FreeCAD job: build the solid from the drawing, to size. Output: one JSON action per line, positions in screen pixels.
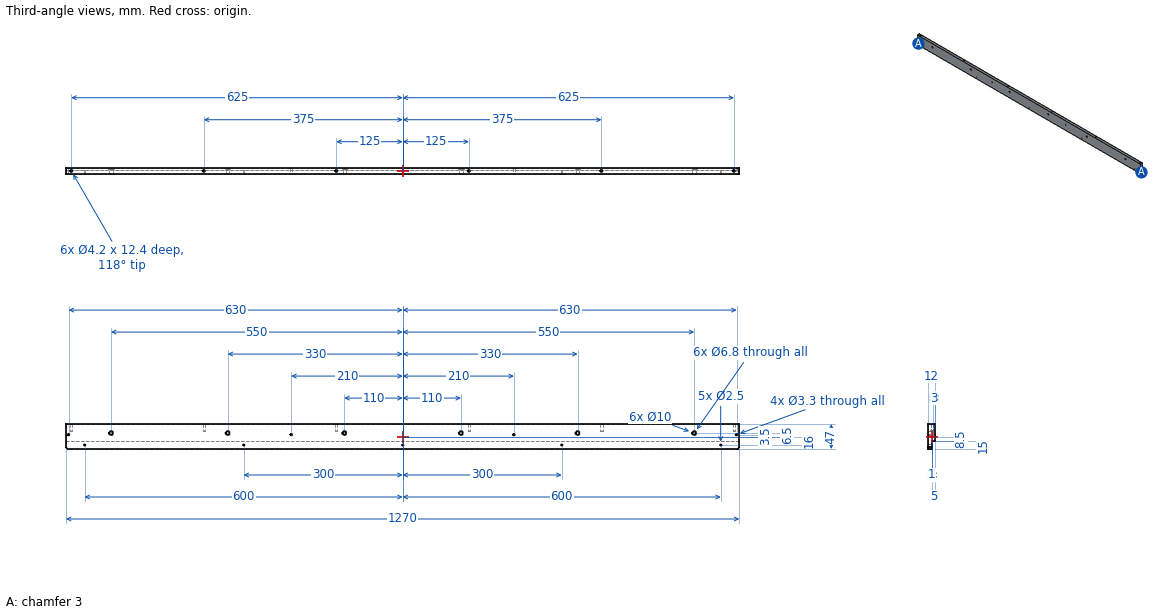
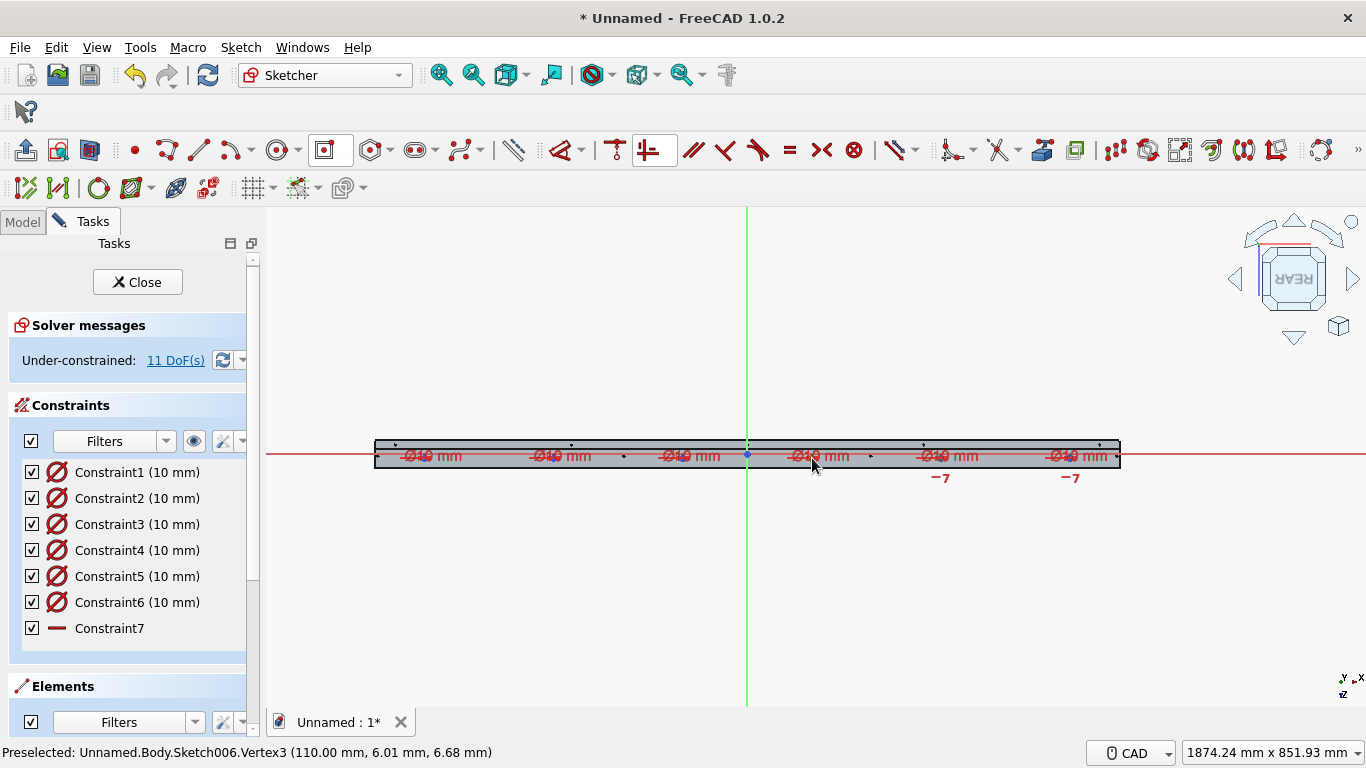
{"action": "key", "text": "h"}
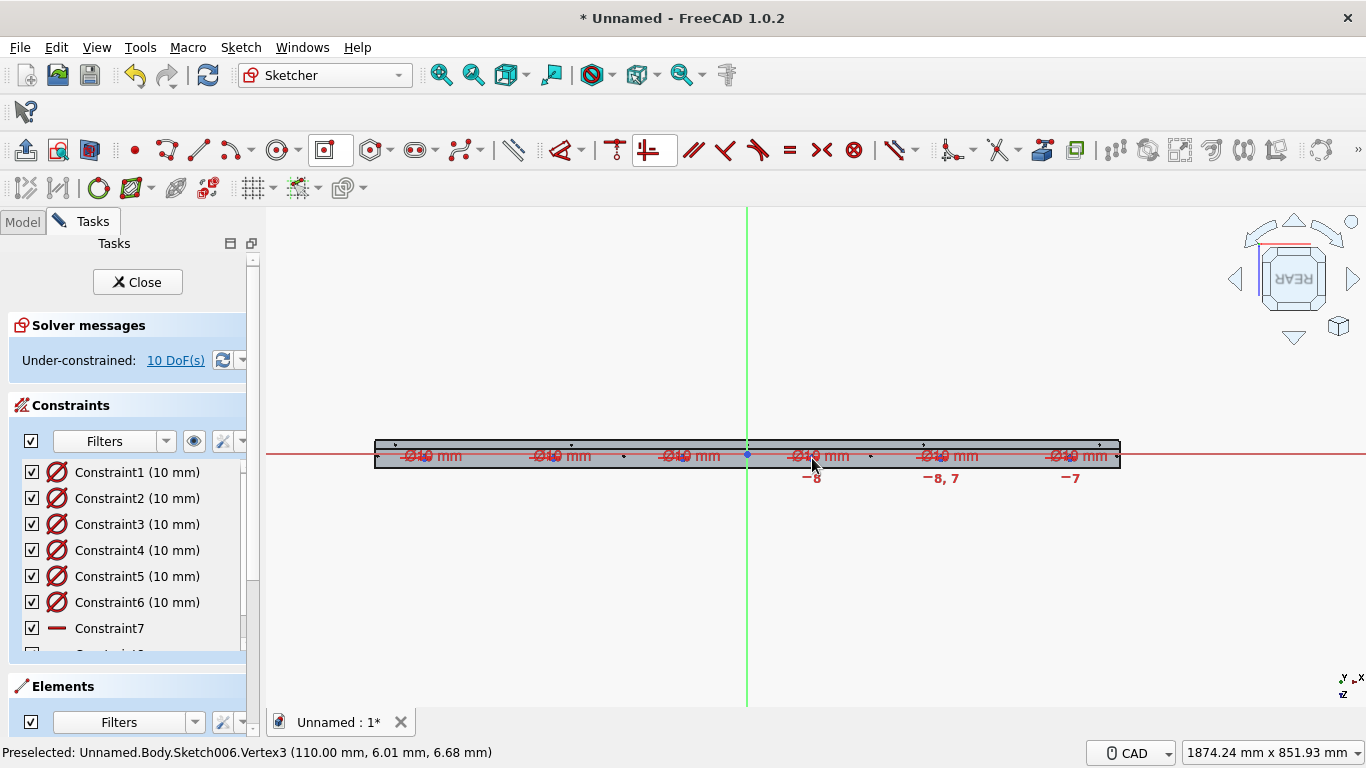
{"action": "left_click", "coordinate": [812, 458]}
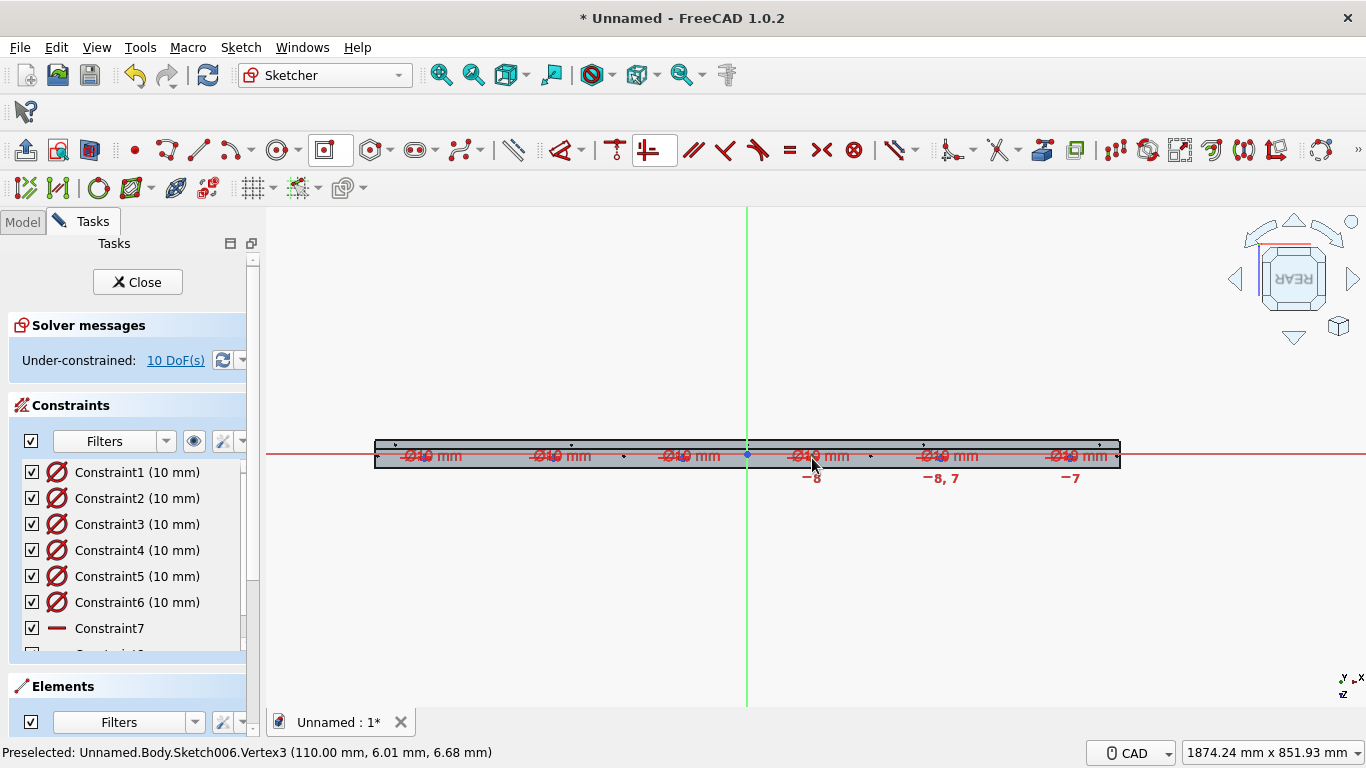
{"action": "left_click", "coordinate": [683, 458]}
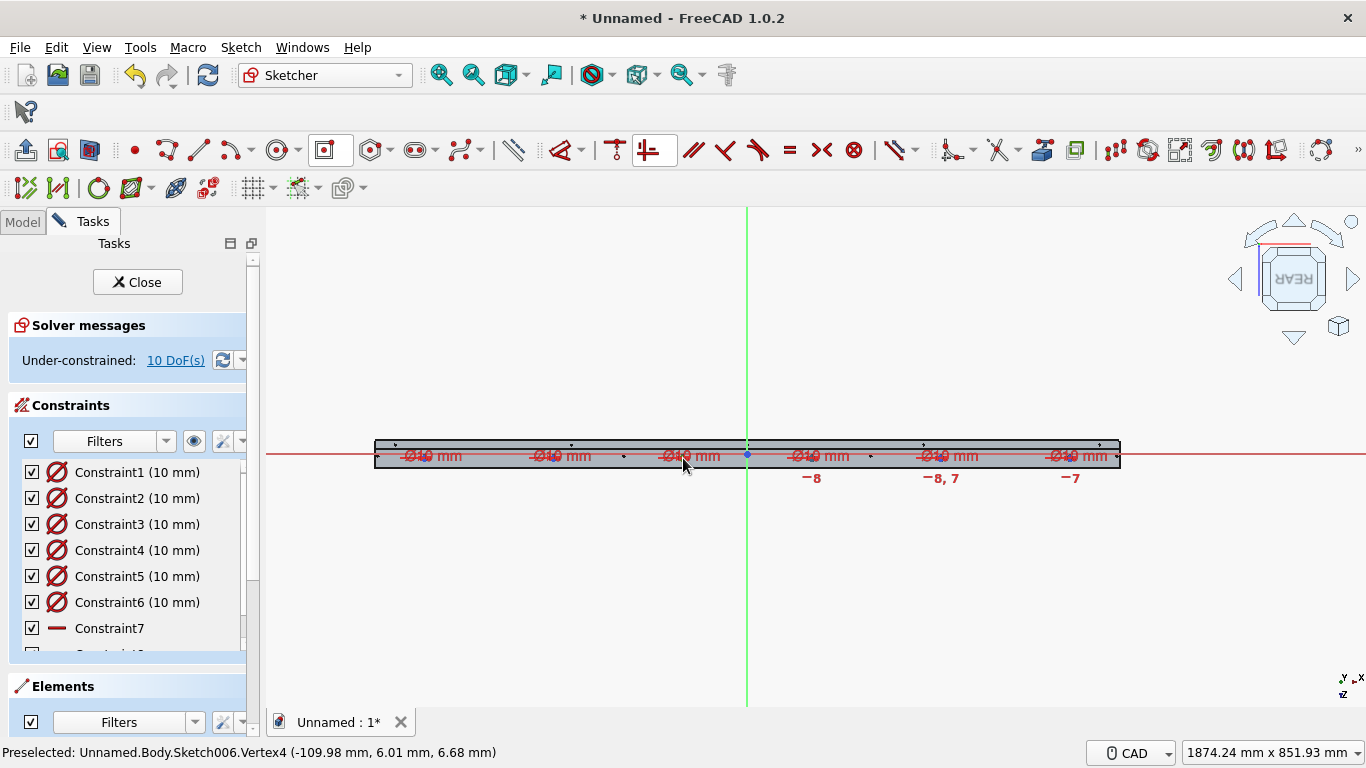
{"action": "left_click", "coordinate": [672, 150]}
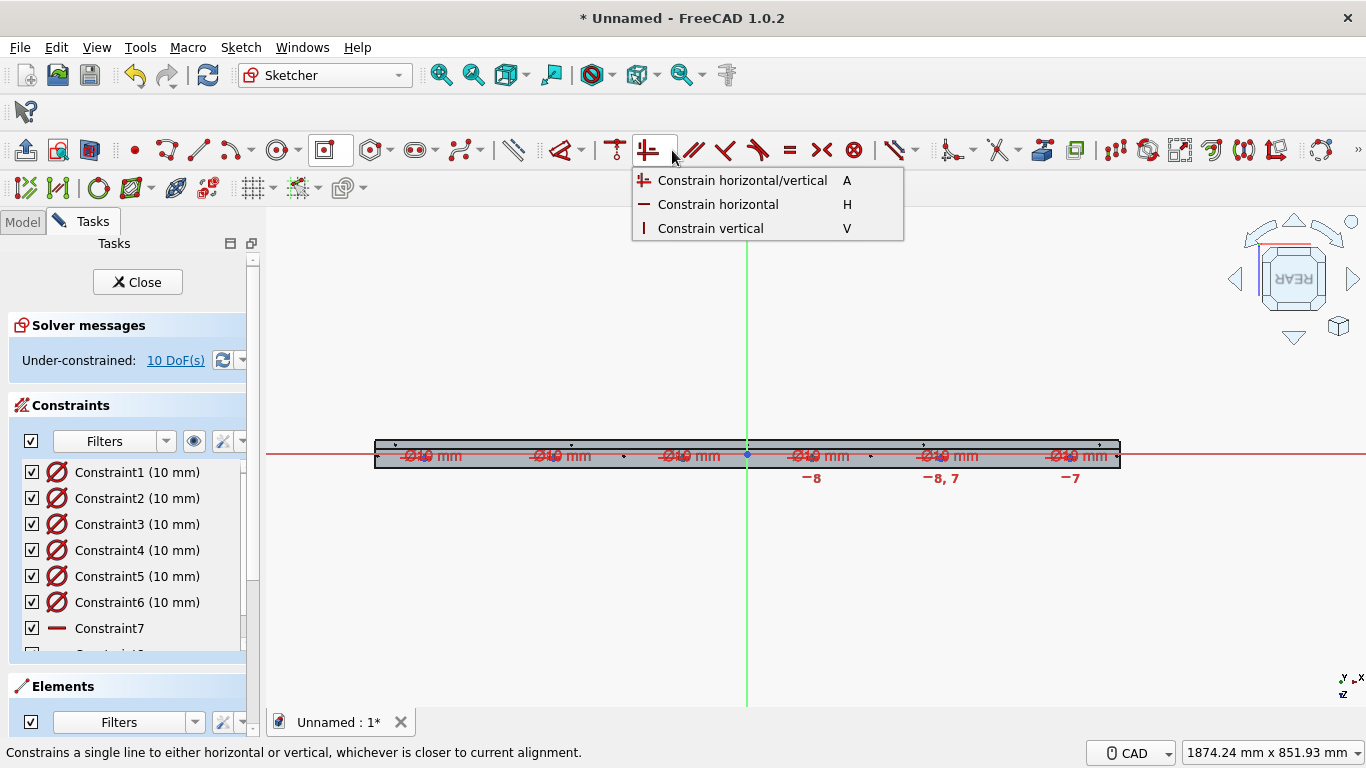
{"action": "left_click", "coordinate": [768, 204]}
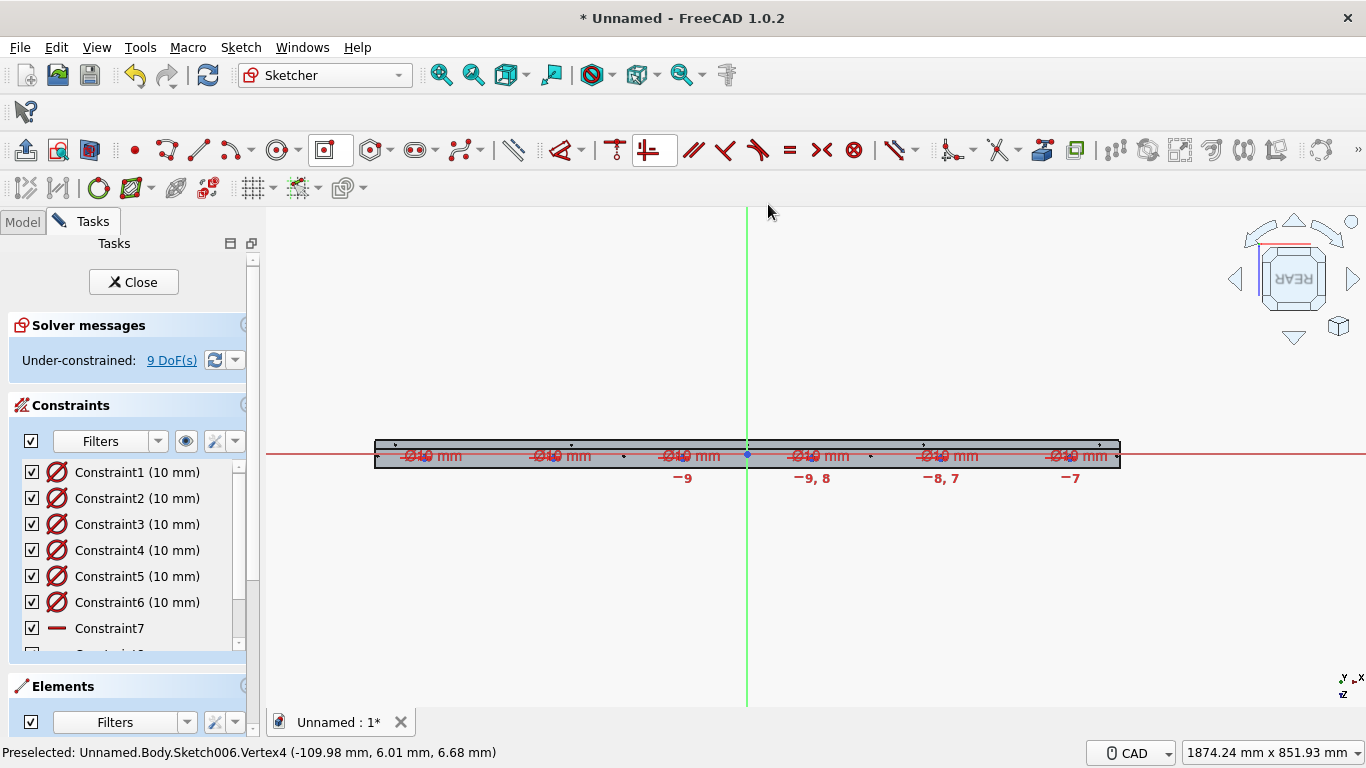
{"action": "left_click", "coordinate": [683, 458]}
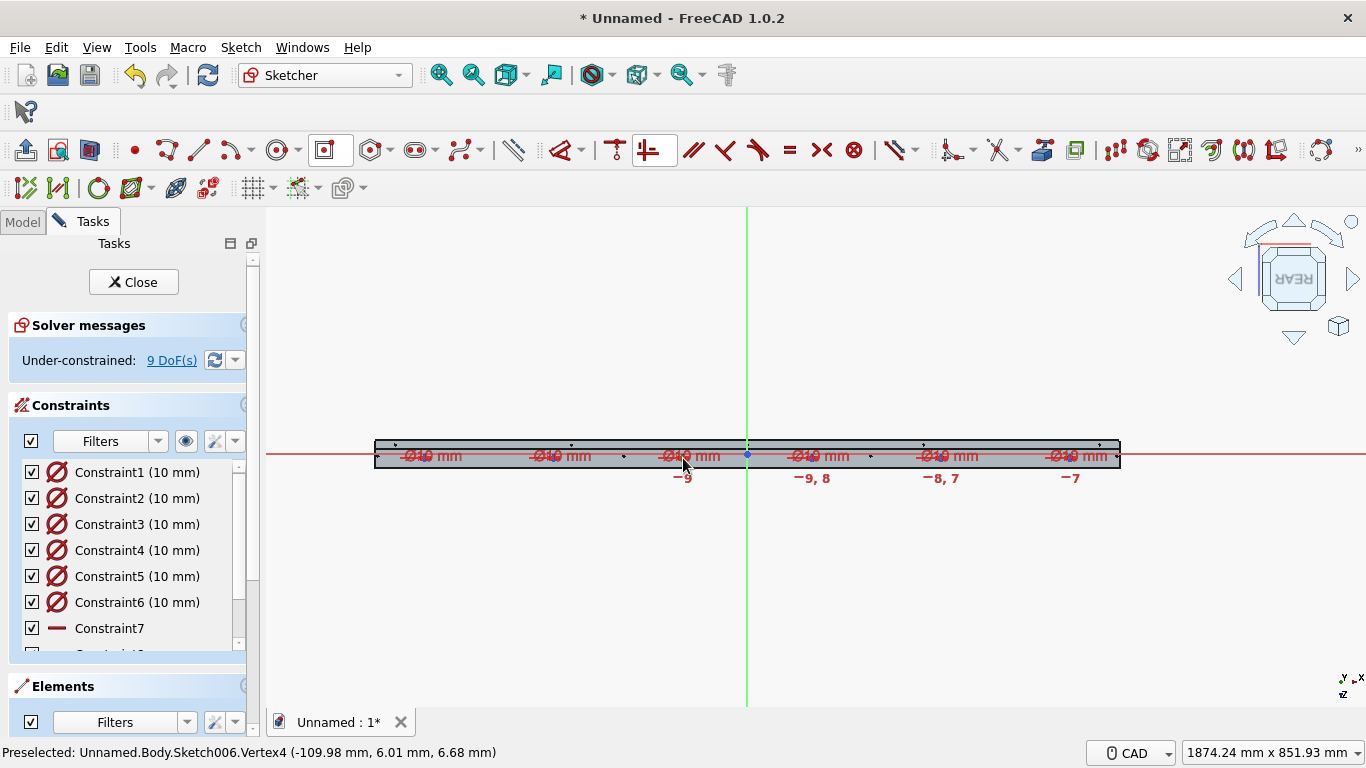
{"action": "left_click", "coordinate": [554, 458]}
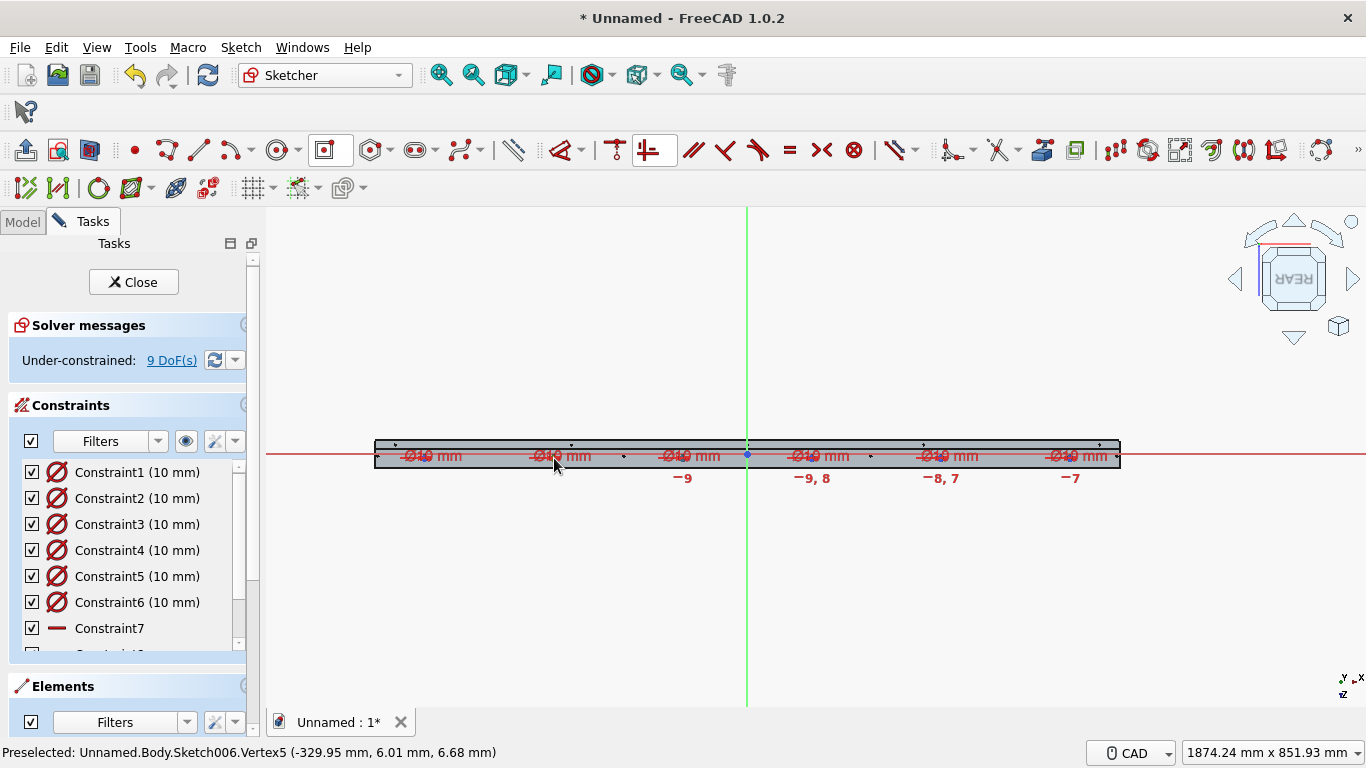
{"action": "key", "text": "h"}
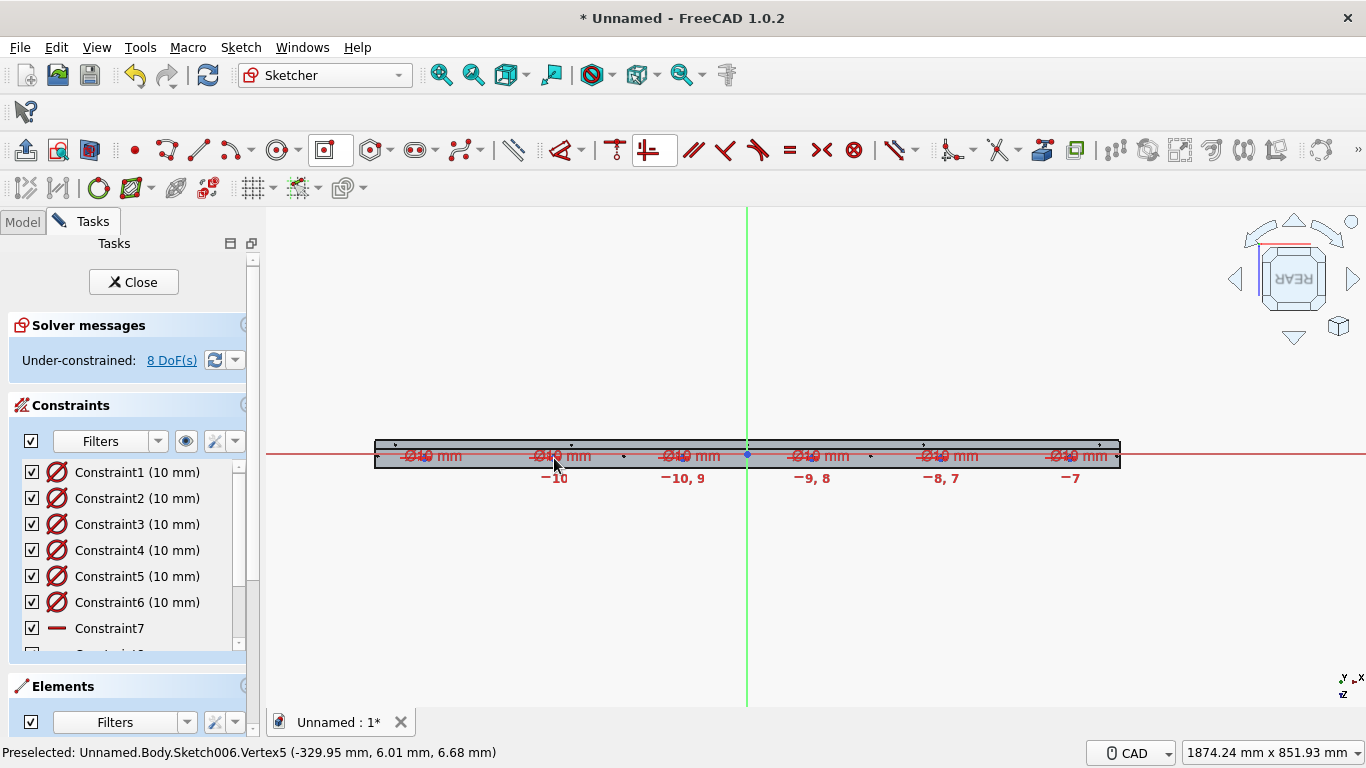
{"action": "left_click", "coordinate": [554, 458]}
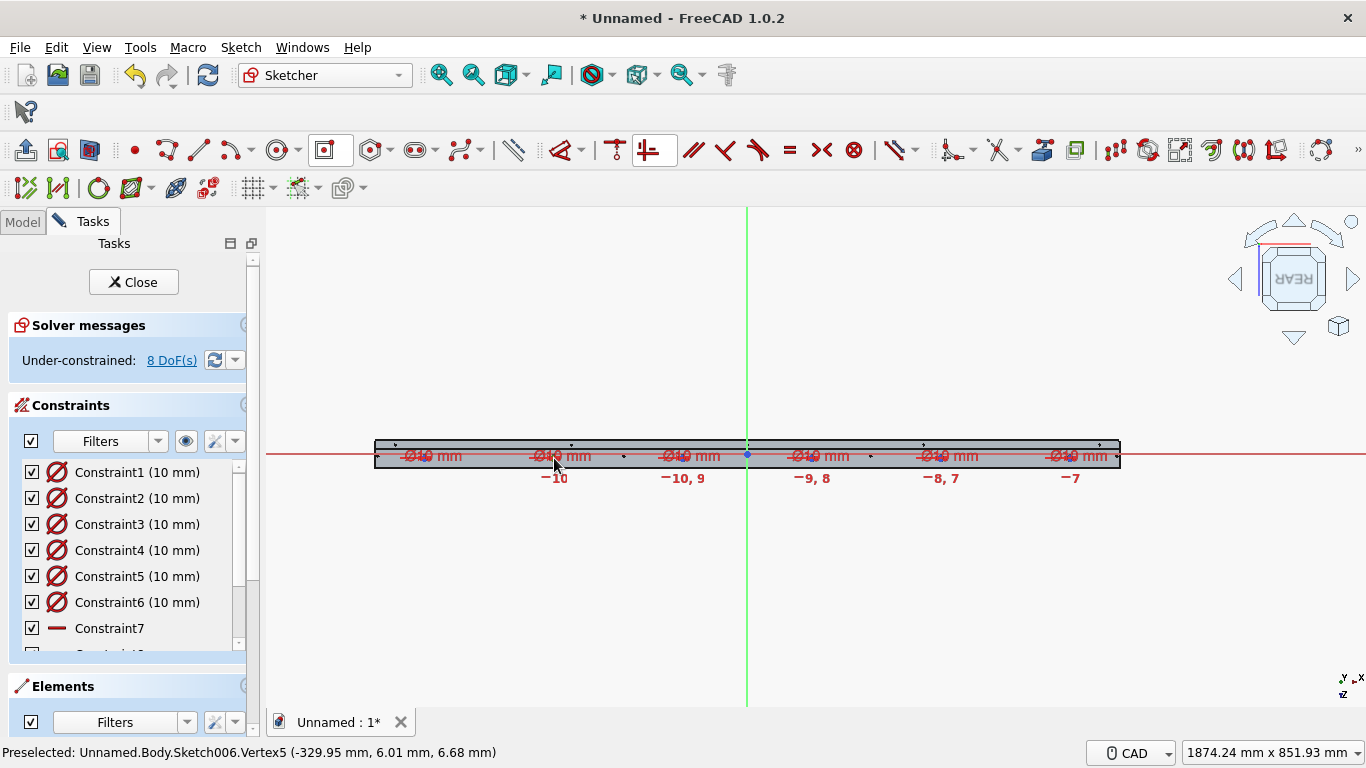
{"action": "left_click", "coordinate": [425, 458]}